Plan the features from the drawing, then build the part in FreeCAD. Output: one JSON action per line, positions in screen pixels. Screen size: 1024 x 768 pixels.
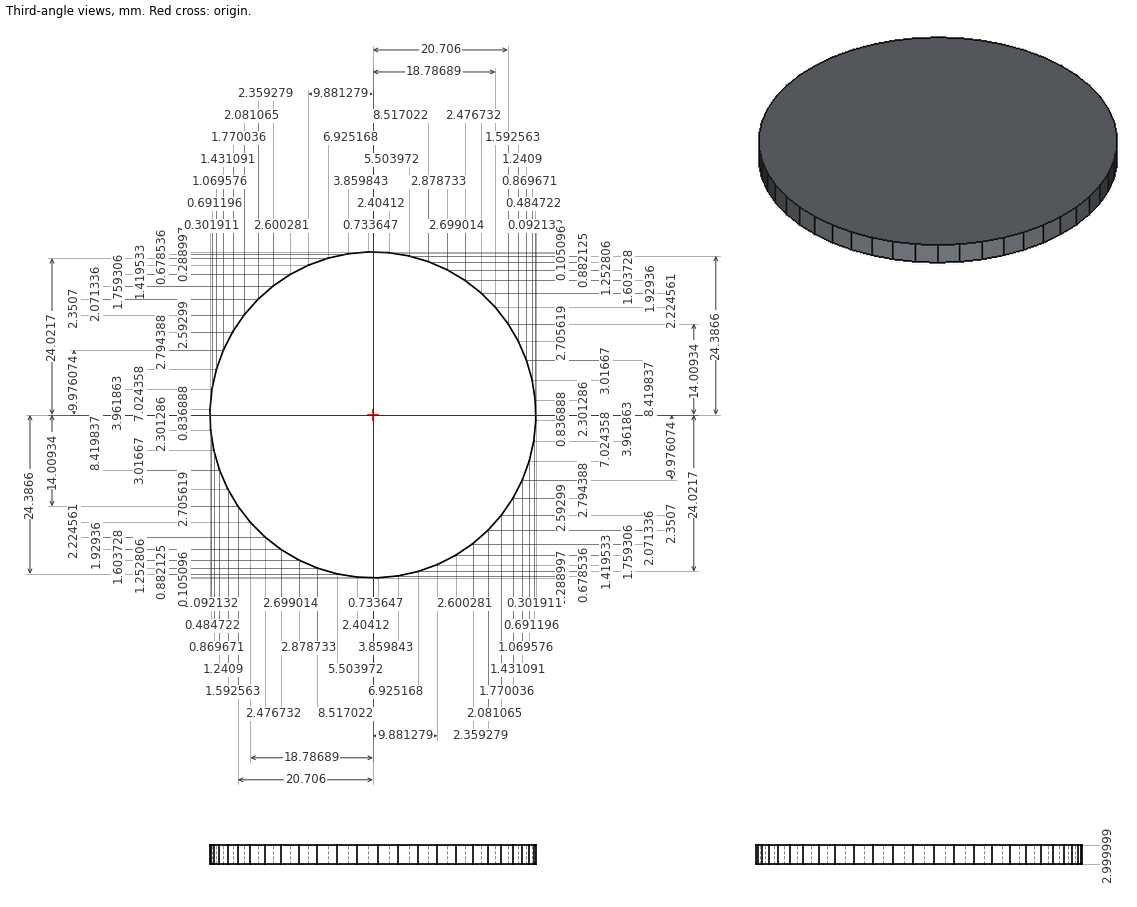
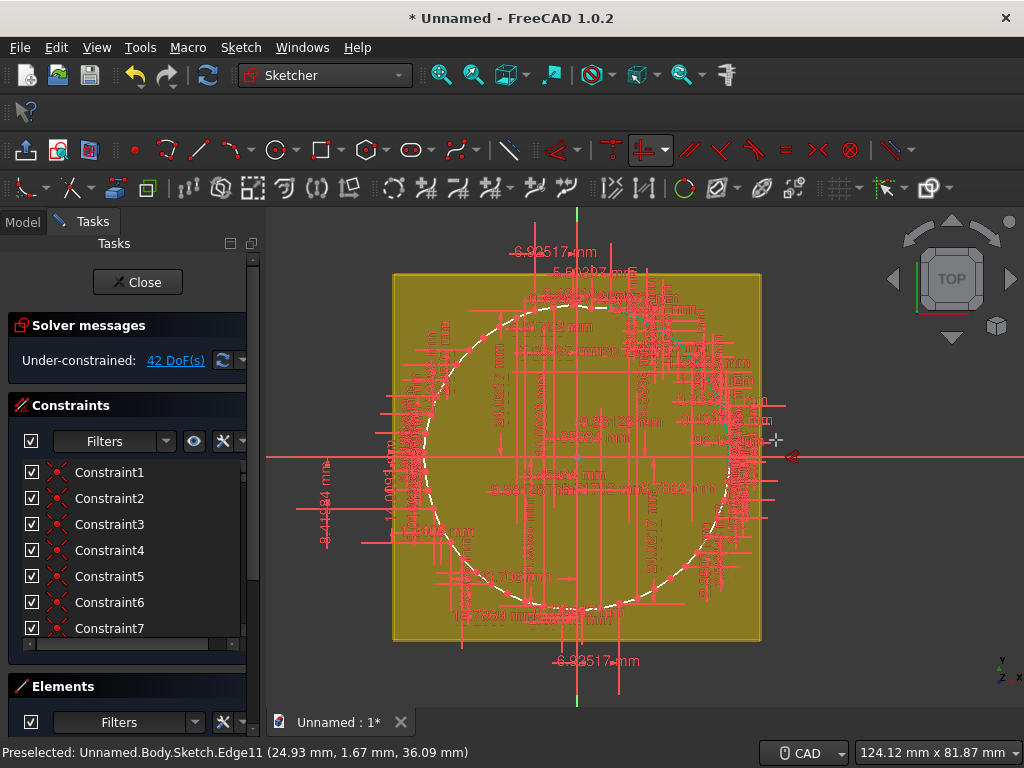
{"action": "scroll", "coordinate": [729, 468], "scroll_direction": "up", "scroll_amount": 16}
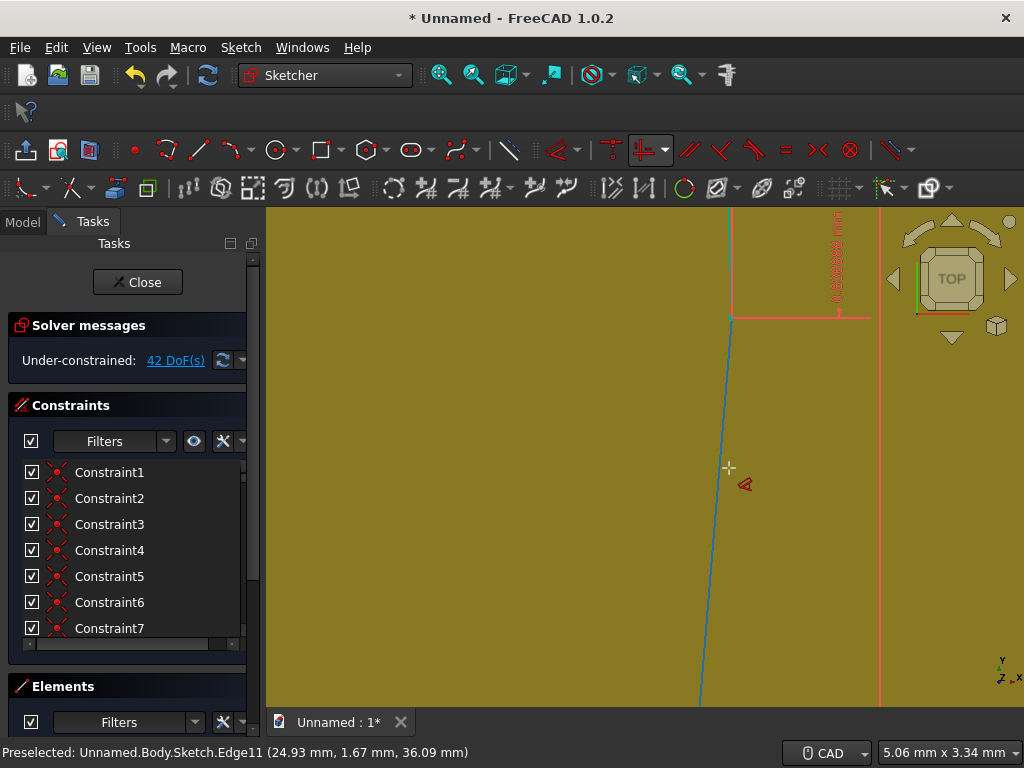
{"action": "left_click", "coordinate": [720, 458]}
{"action": "left_click", "coordinate": [712, 284]}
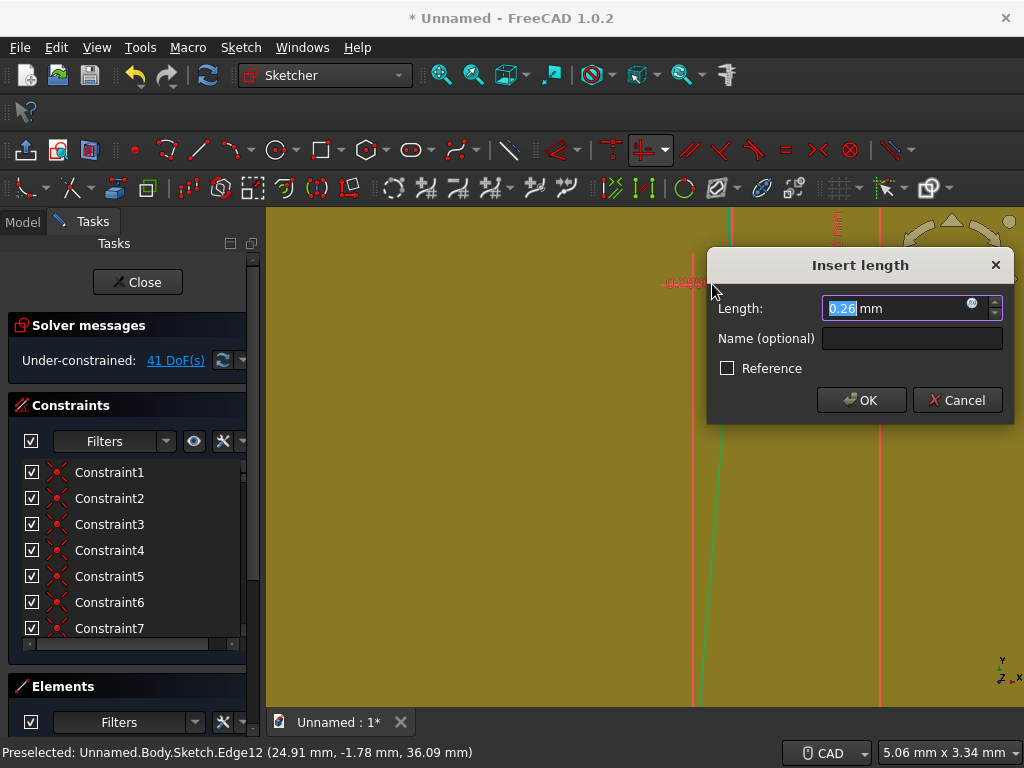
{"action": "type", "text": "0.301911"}
{"action": "key", "text": "Return"}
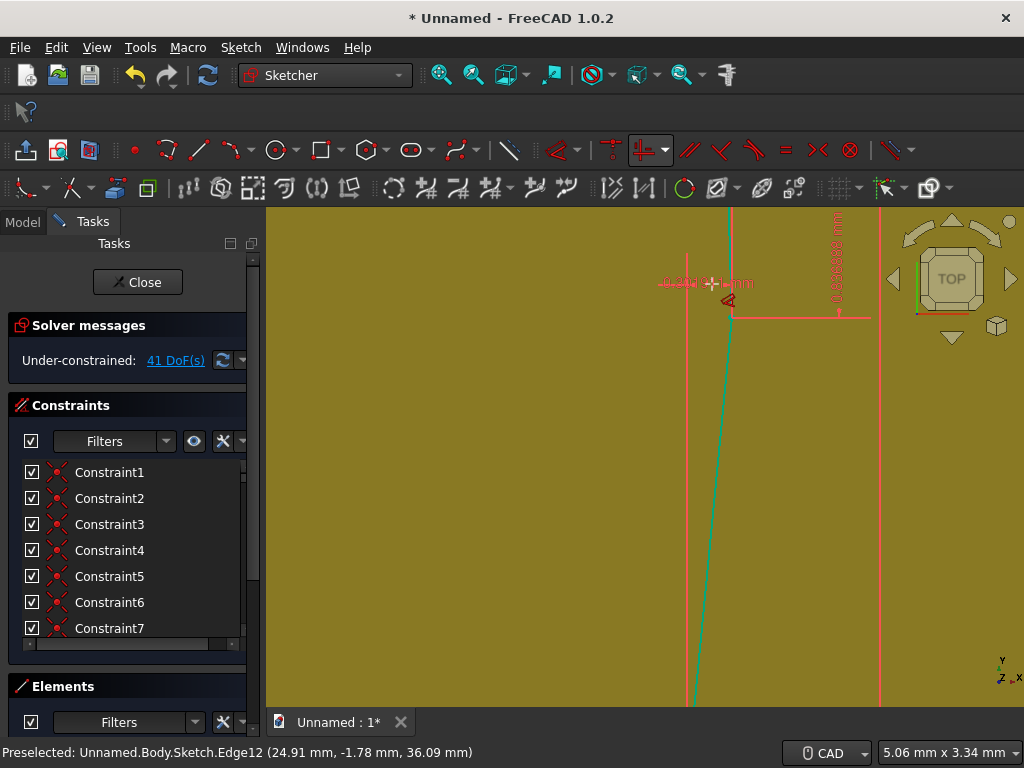
{"action": "scroll", "coordinate": [764, 471], "scroll_direction": "down", "scroll_amount": 15}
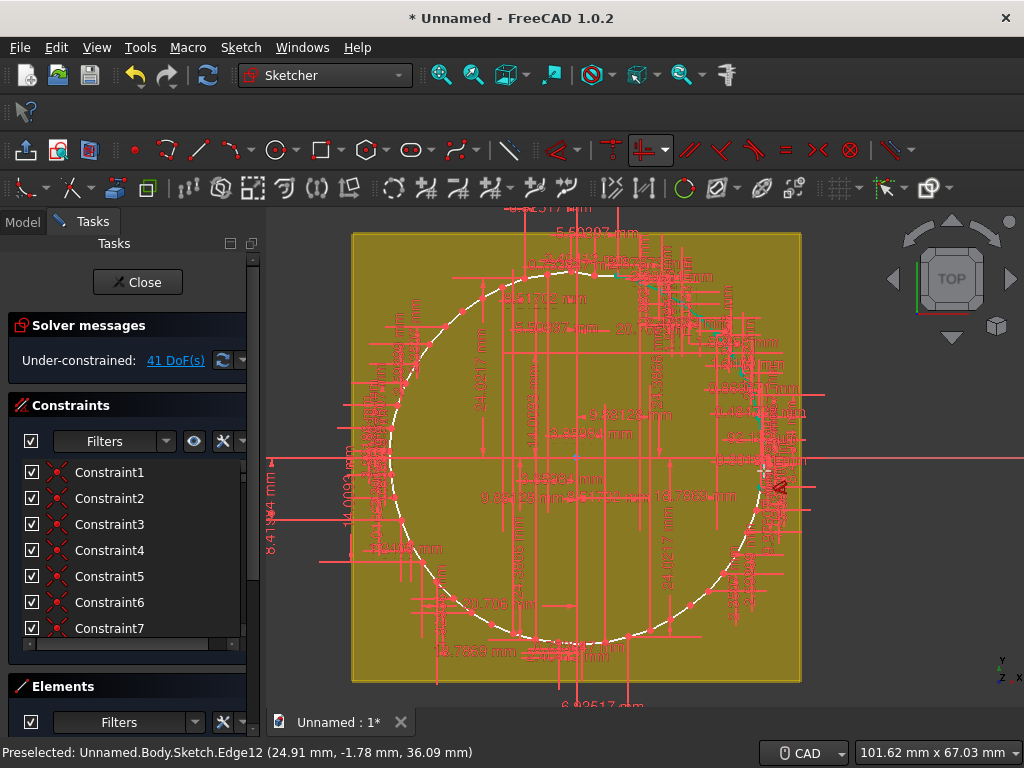
{"action": "scroll", "coordinate": [759, 494], "scroll_direction": "up", "scroll_amount": 11}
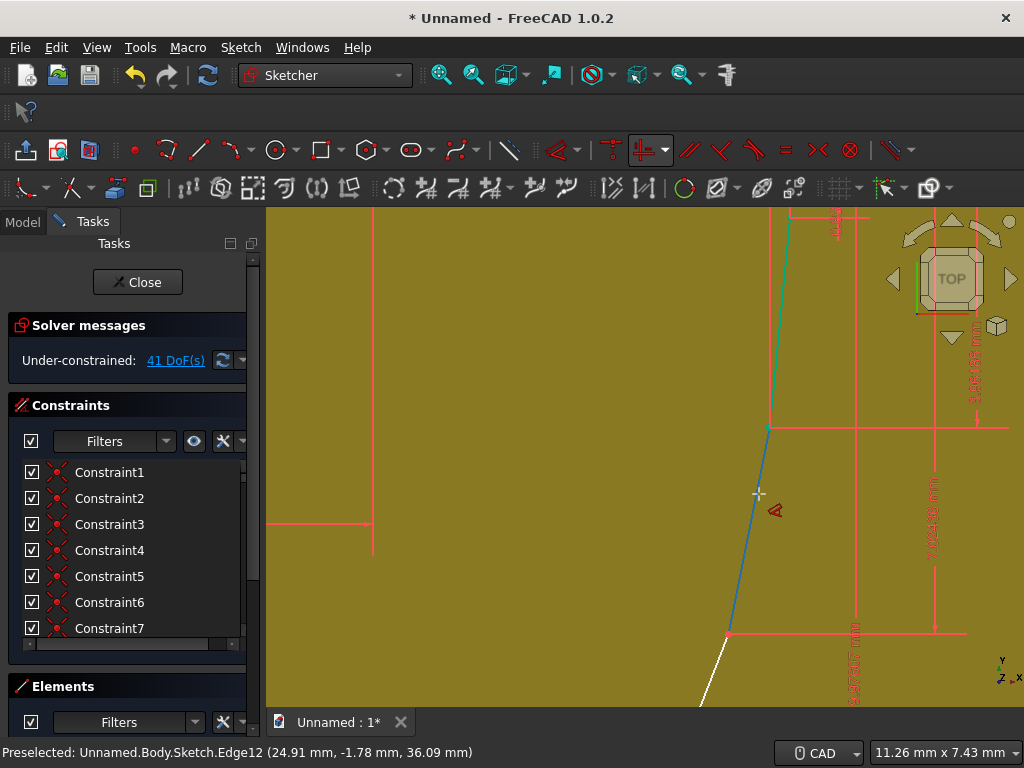
{"action": "left_click", "coordinate": [757, 490]}
{"action": "left_click", "coordinate": [749, 668]}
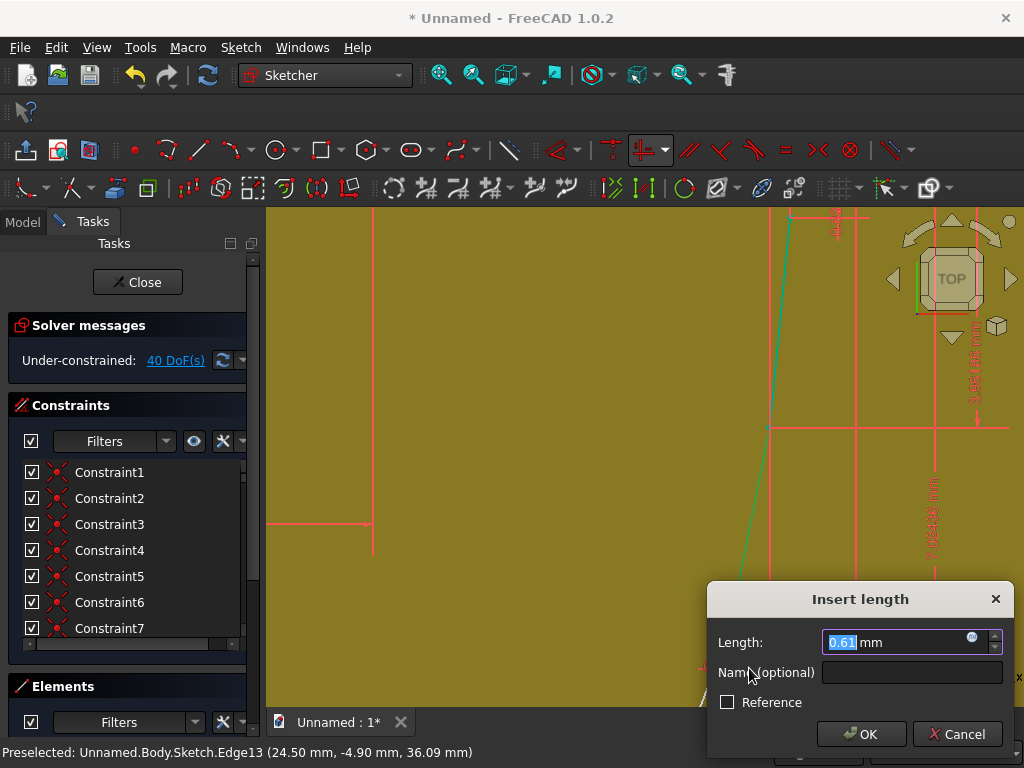
{"action": "type", "text": "0.691196"}
{"action": "key", "text": "Return"}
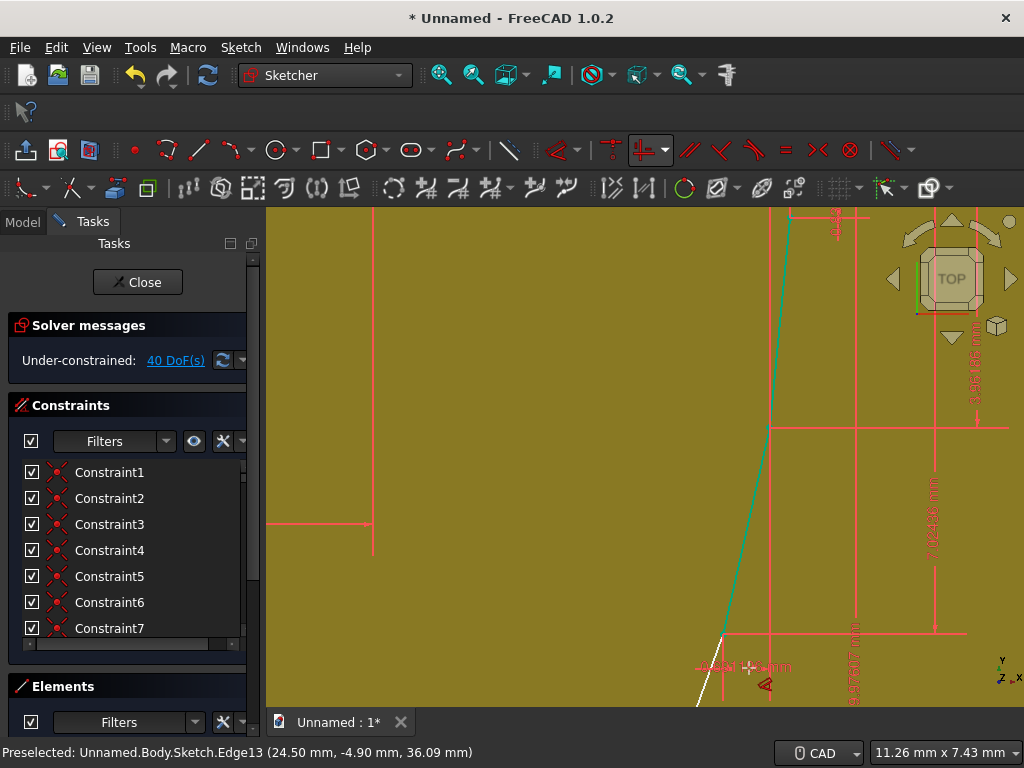
{"action": "left_click", "coordinate": [709, 674]}
{"action": "left_click", "coordinate": [687, 600]}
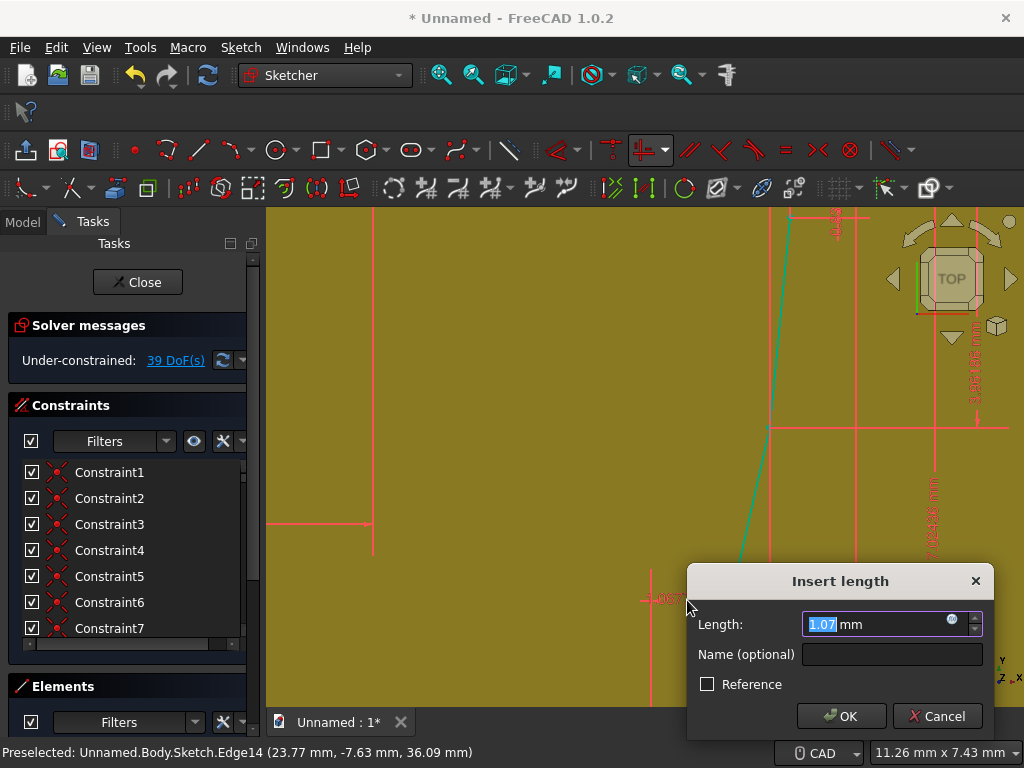
{"action": "type", "text": "1.069576"}
{"action": "key", "text": "Return"}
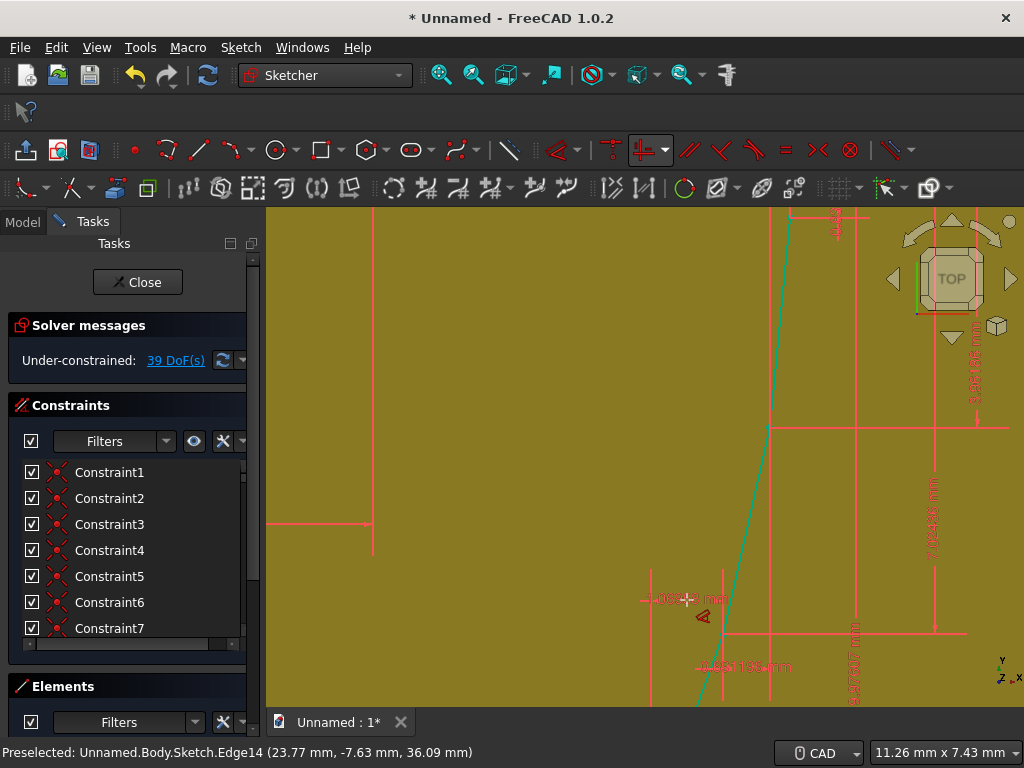
{"action": "scroll", "coordinate": [723, 487], "scroll_direction": "down", "scroll_amount": 12}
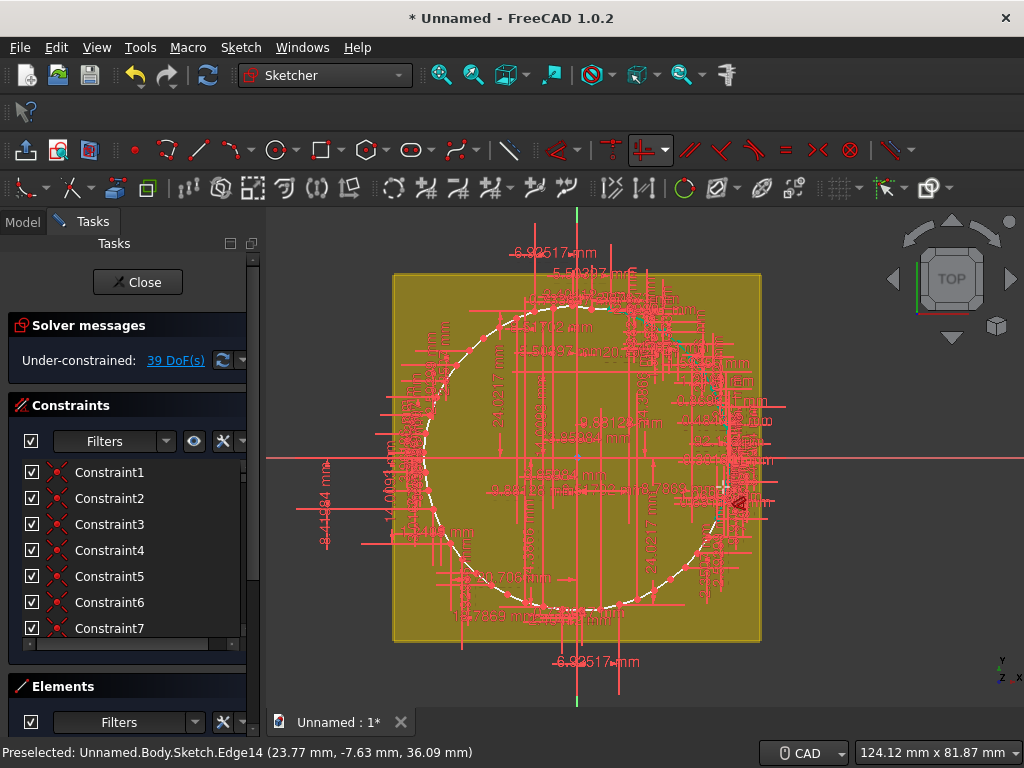
{"action": "scroll", "coordinate": [714, 524], "scroll_direction": "up", "scroll_amount": 8}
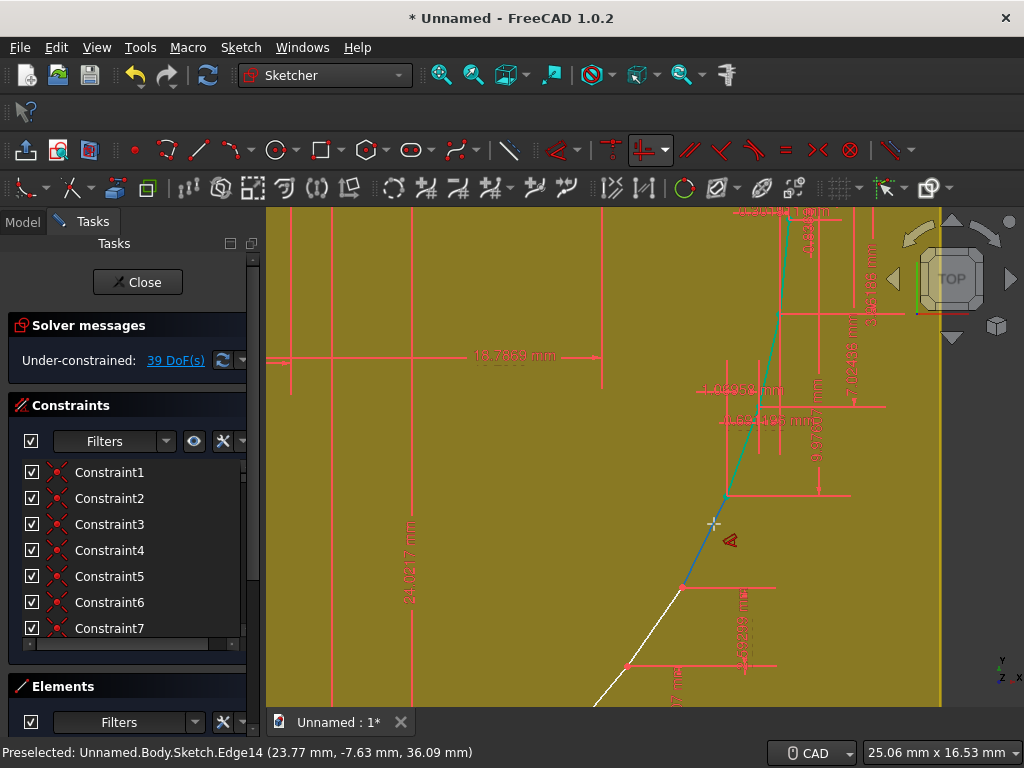
{"action": "left_click", "coordinate": [713, 524]}
{"action": "left_click", "coordinate": [704, 462]}